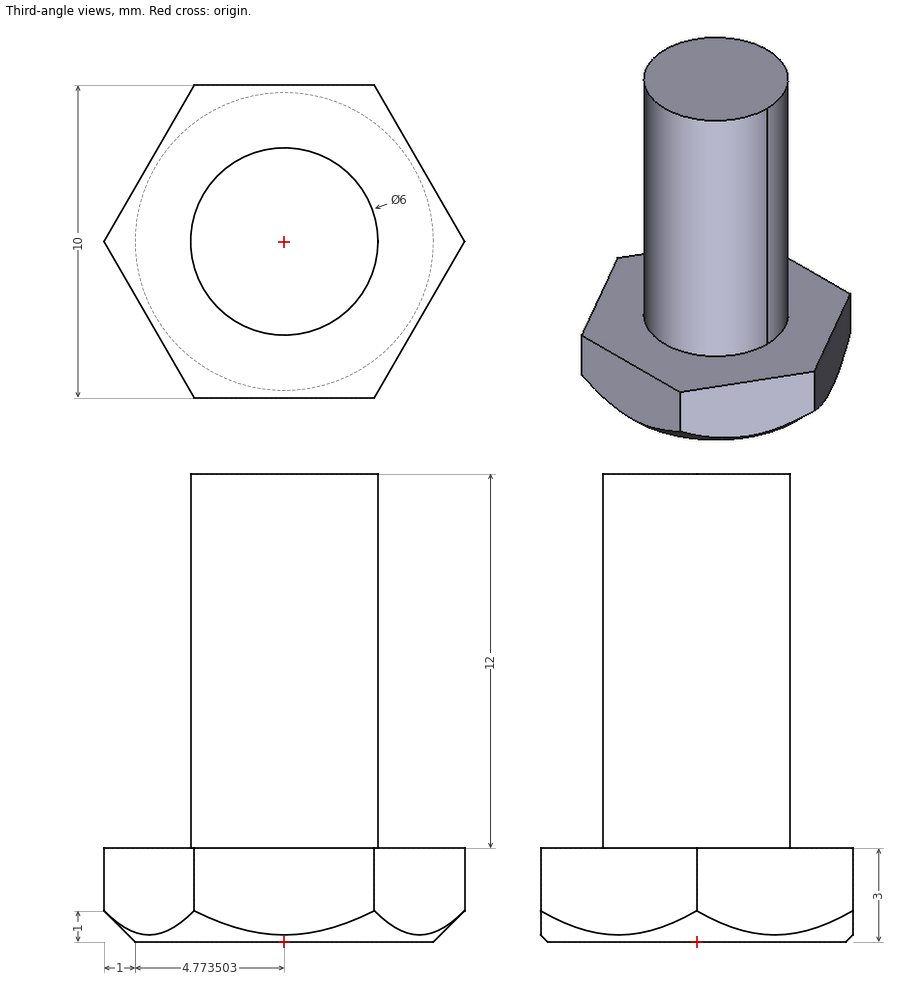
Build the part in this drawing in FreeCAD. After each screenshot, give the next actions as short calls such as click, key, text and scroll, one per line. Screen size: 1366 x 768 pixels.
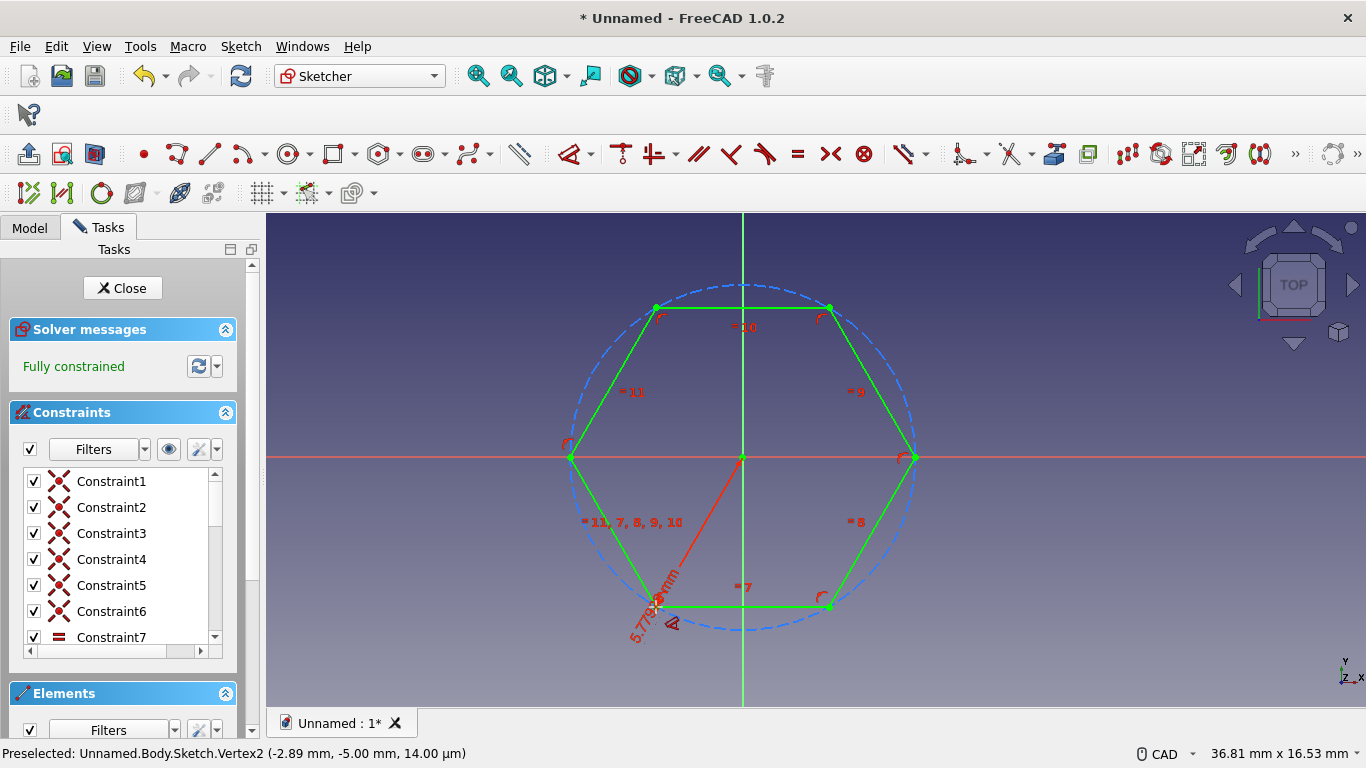
click(829, 308)
click(911, 353)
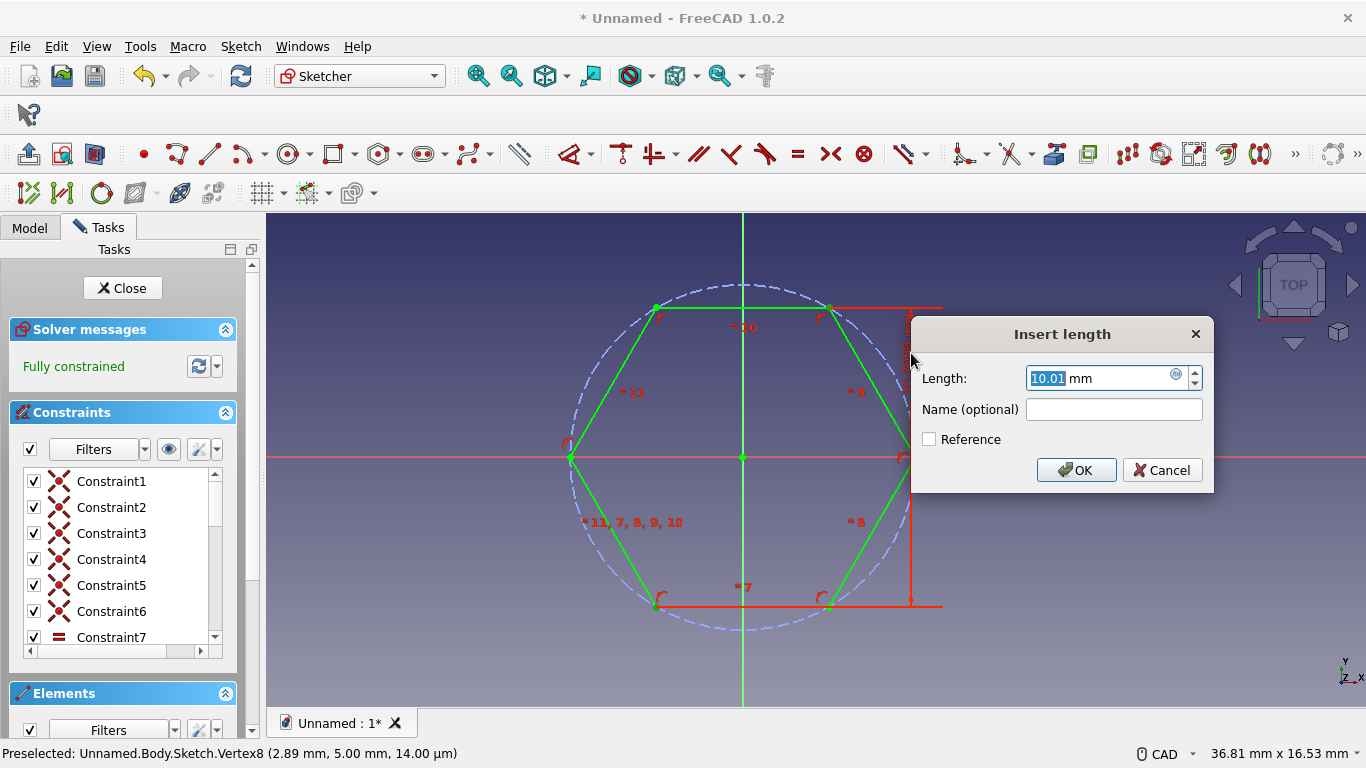
text(10)
key(Return)
key(Escape)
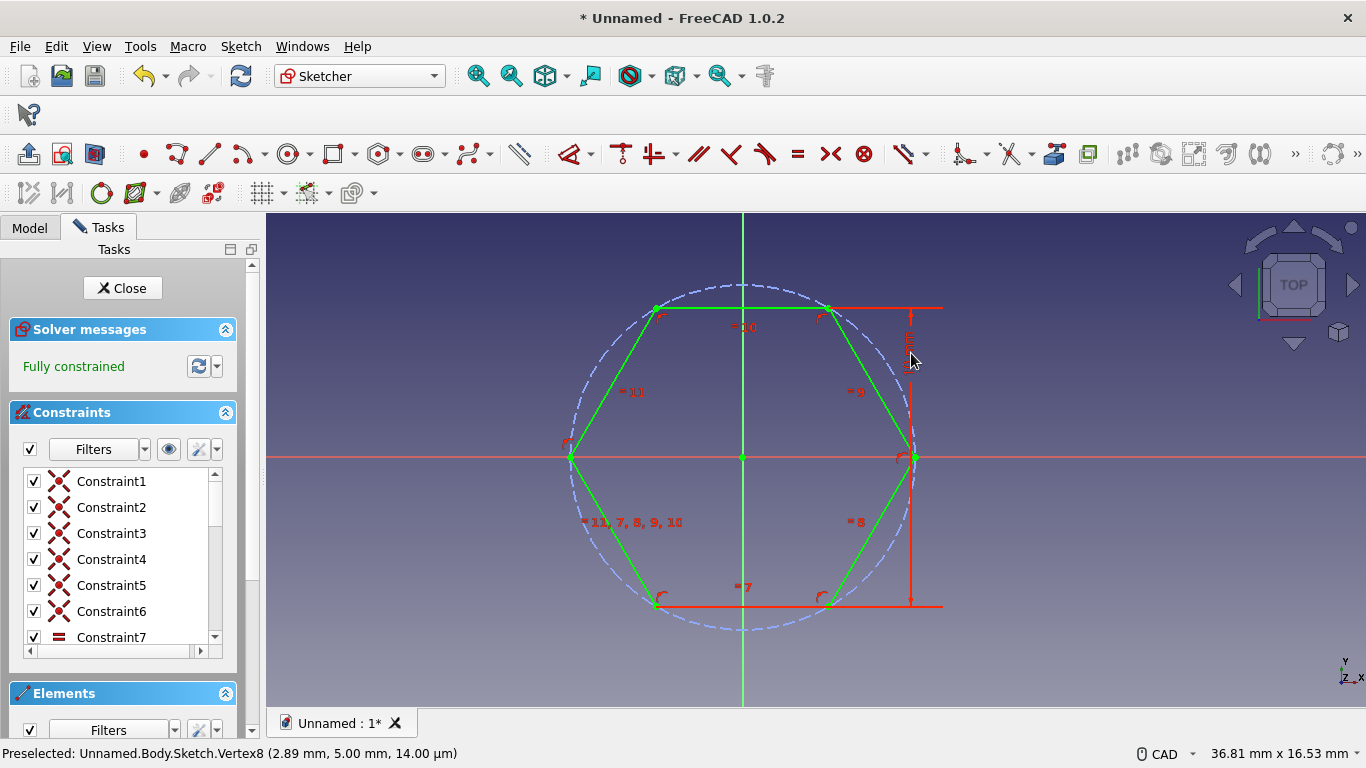
click(123, 288)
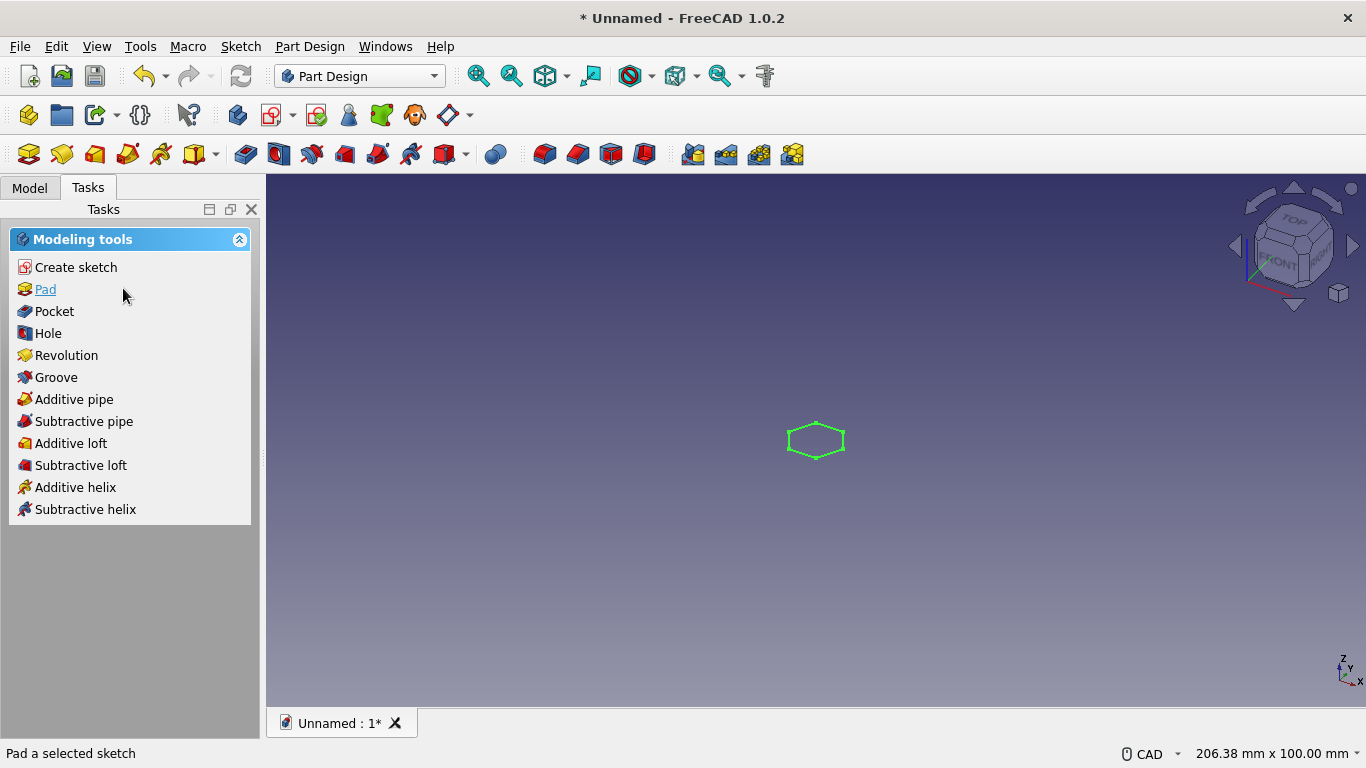
click(29, 154)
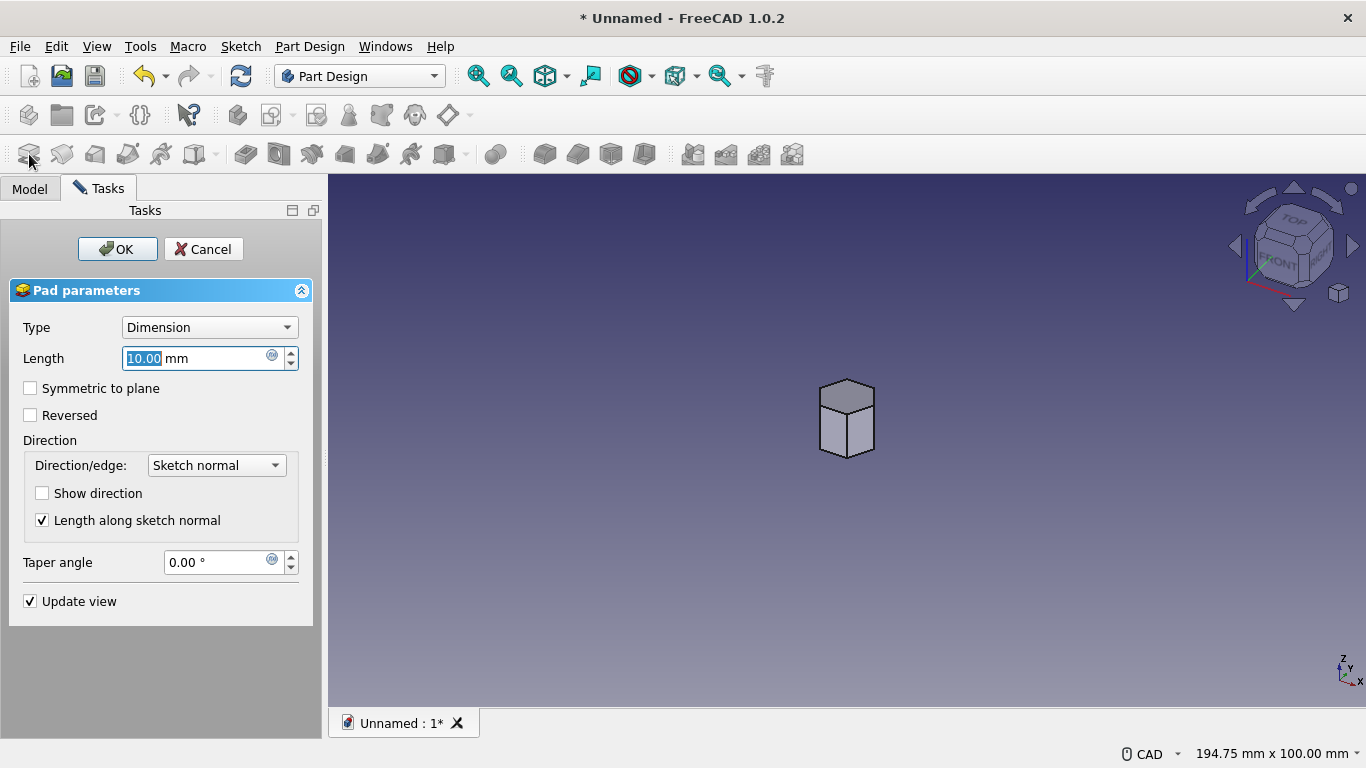
text(3)
key(Tab)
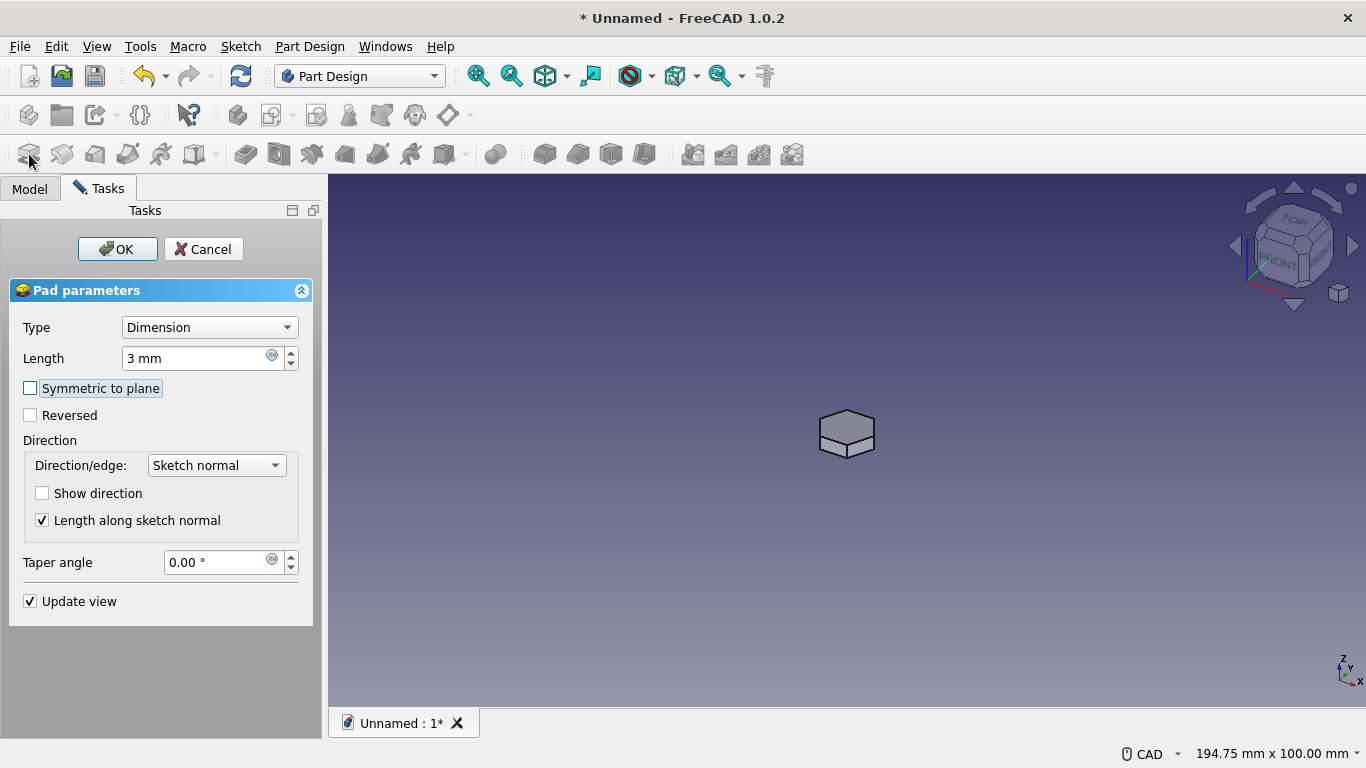
click(118, 249)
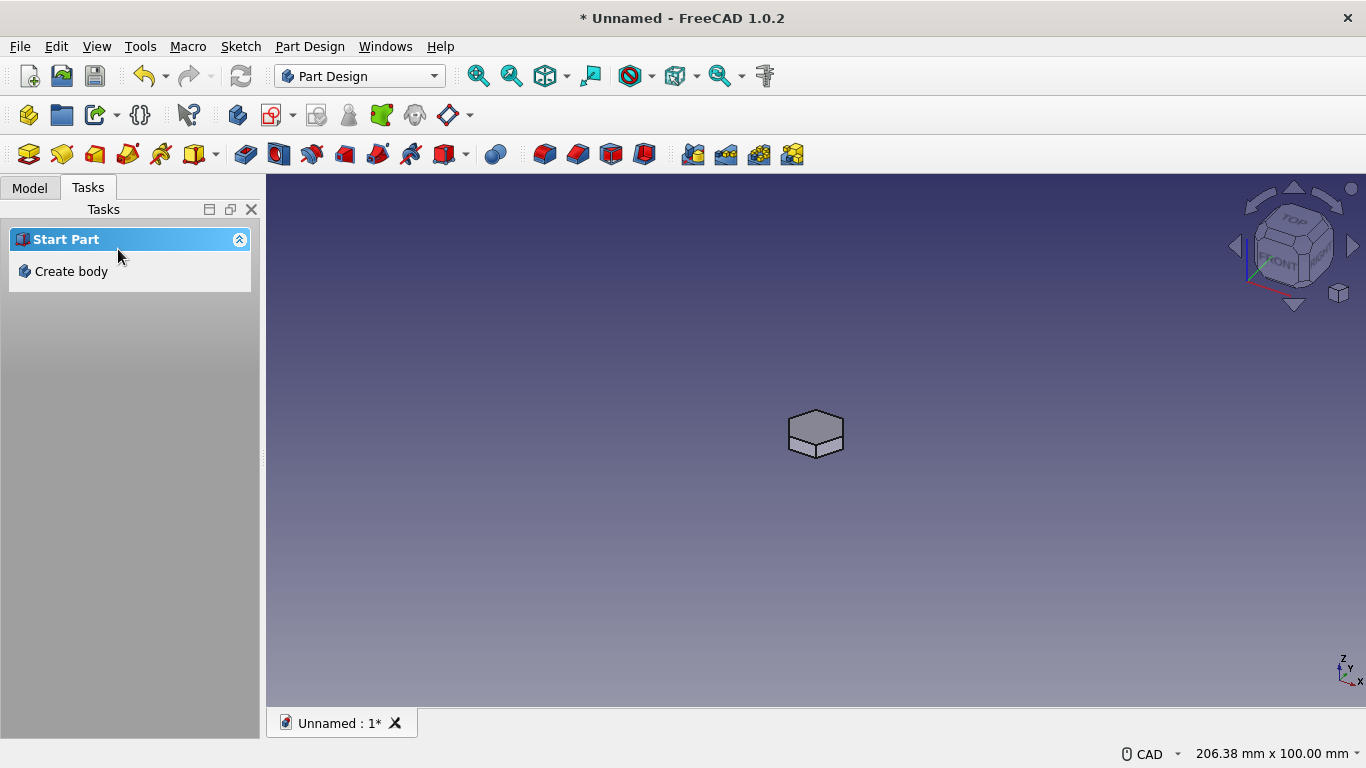
click(479, 76)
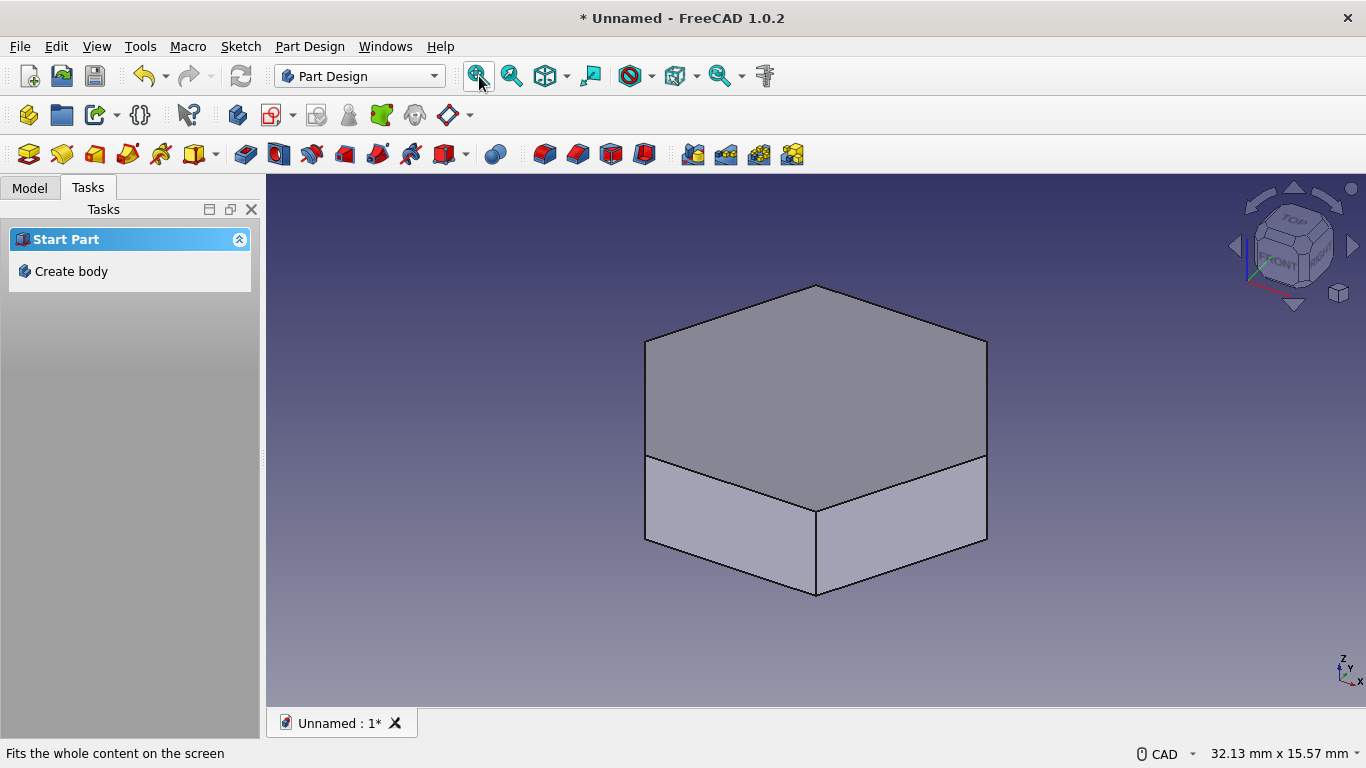
click(816, 397)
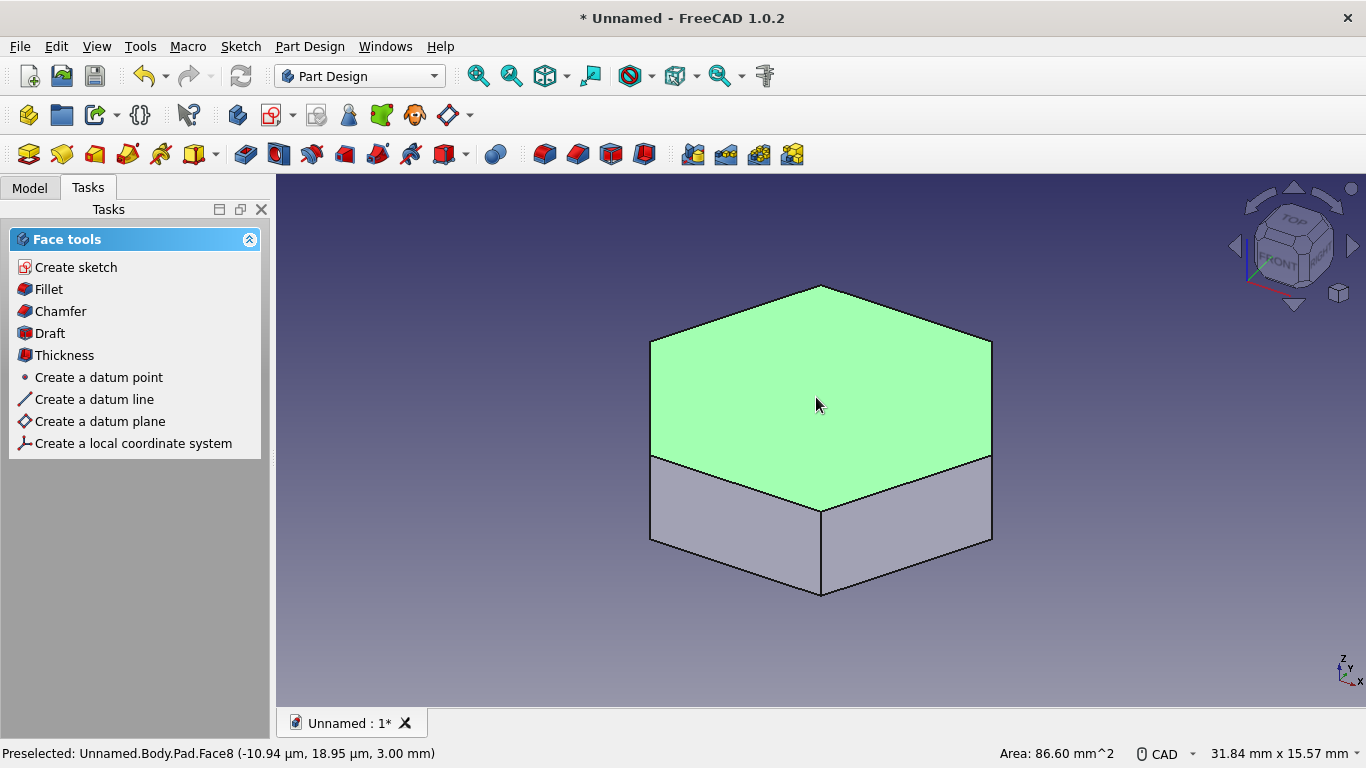
click(270, 116)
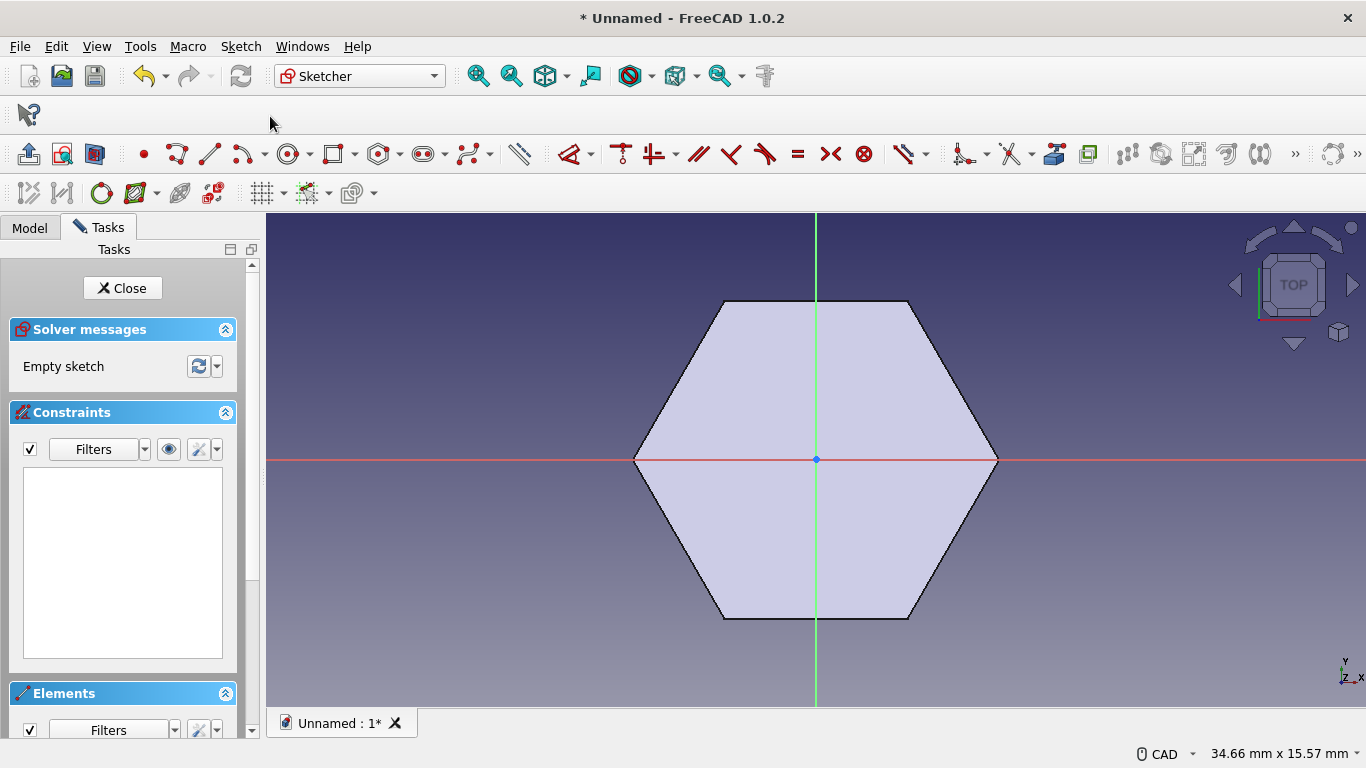
scroll(955, 460, up, 2)